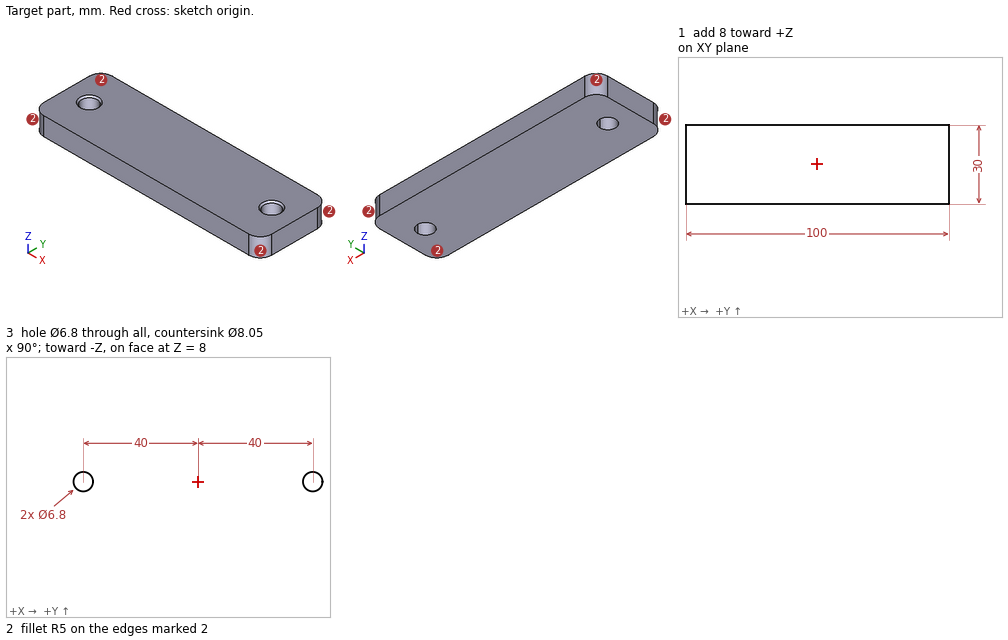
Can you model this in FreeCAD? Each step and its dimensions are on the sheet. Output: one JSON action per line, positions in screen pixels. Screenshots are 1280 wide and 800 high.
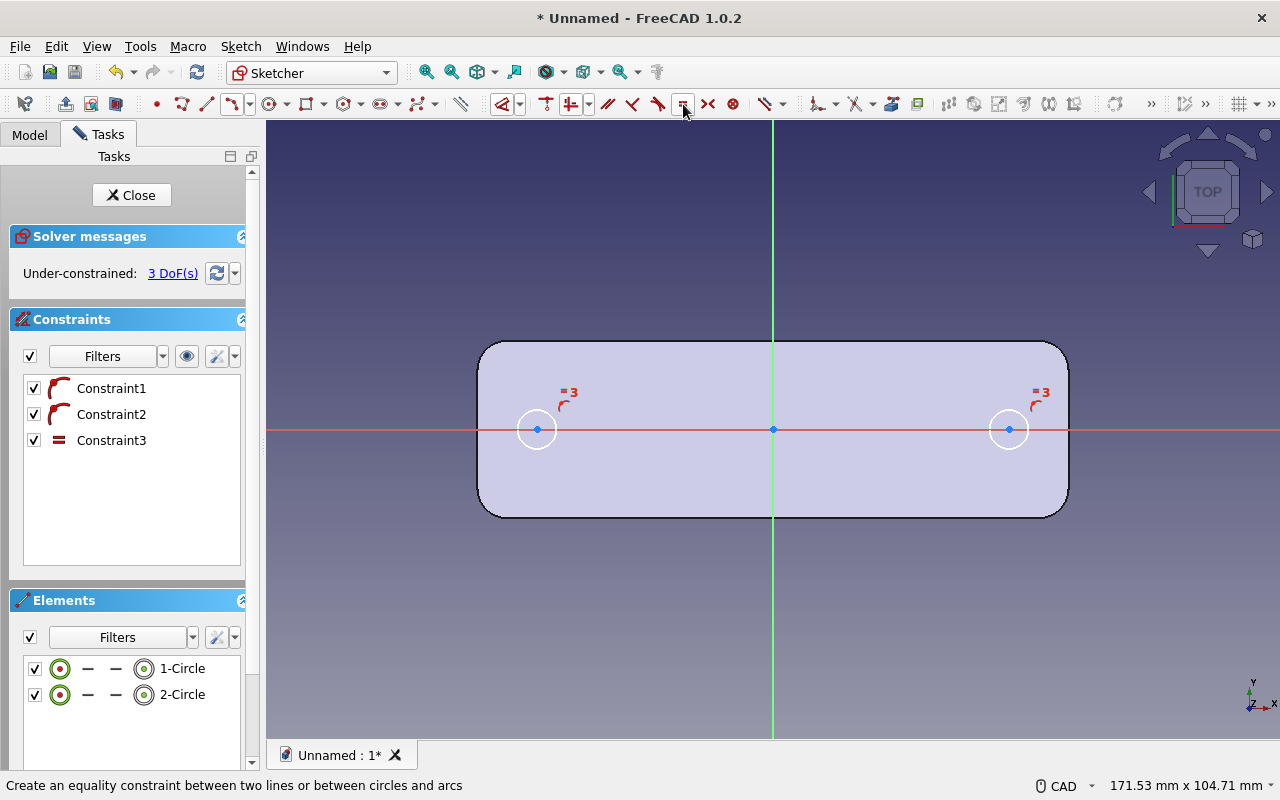
{"action": "left_click", "coordinate": [551, 416]}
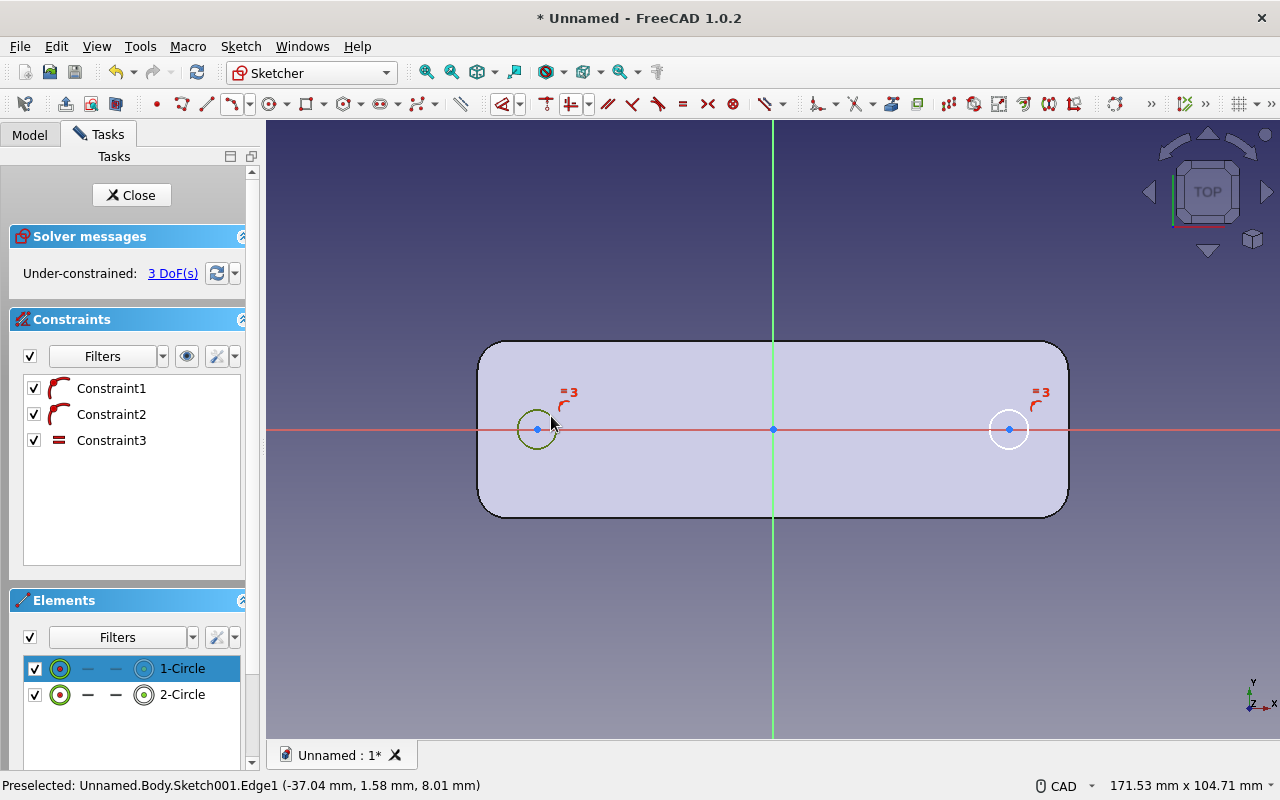
{"action": "key", "text": "k o"}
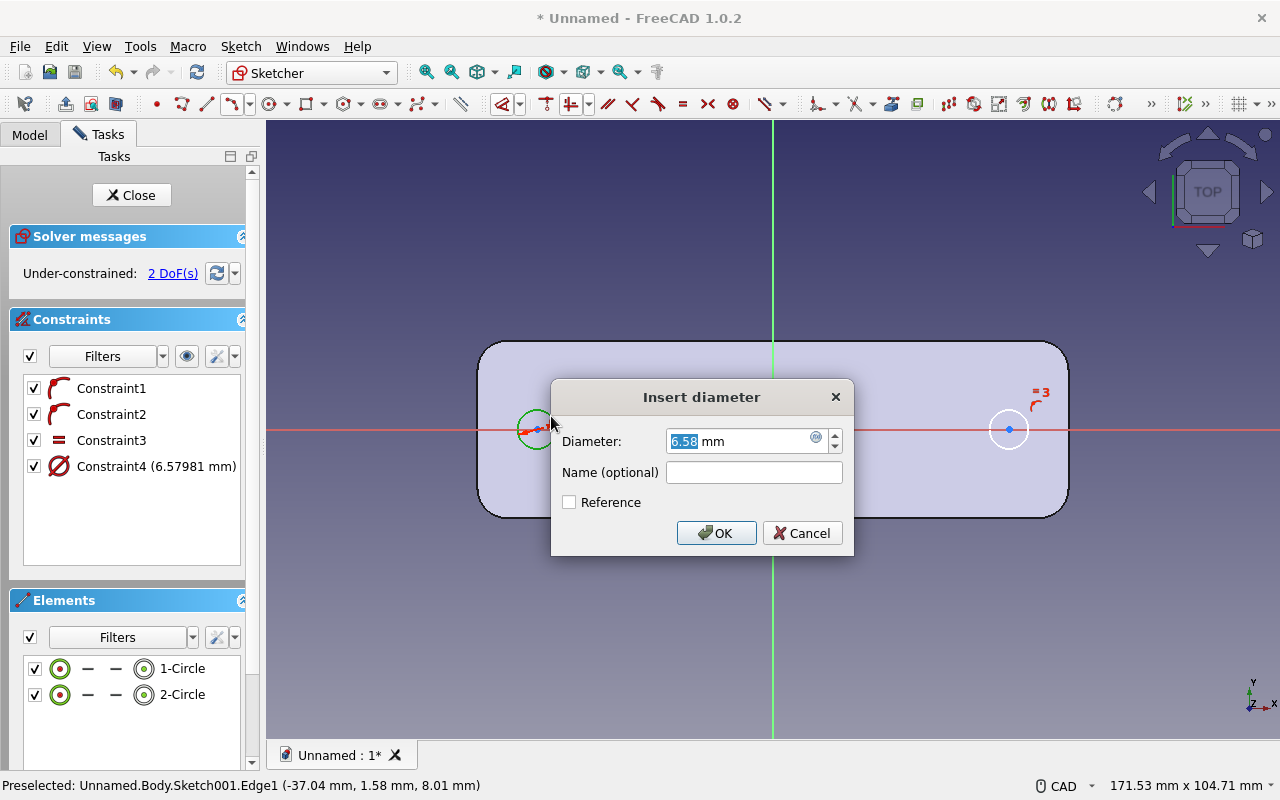
{"action": "type", "text": "6.8"}
{"action": "key", "text": "Return"}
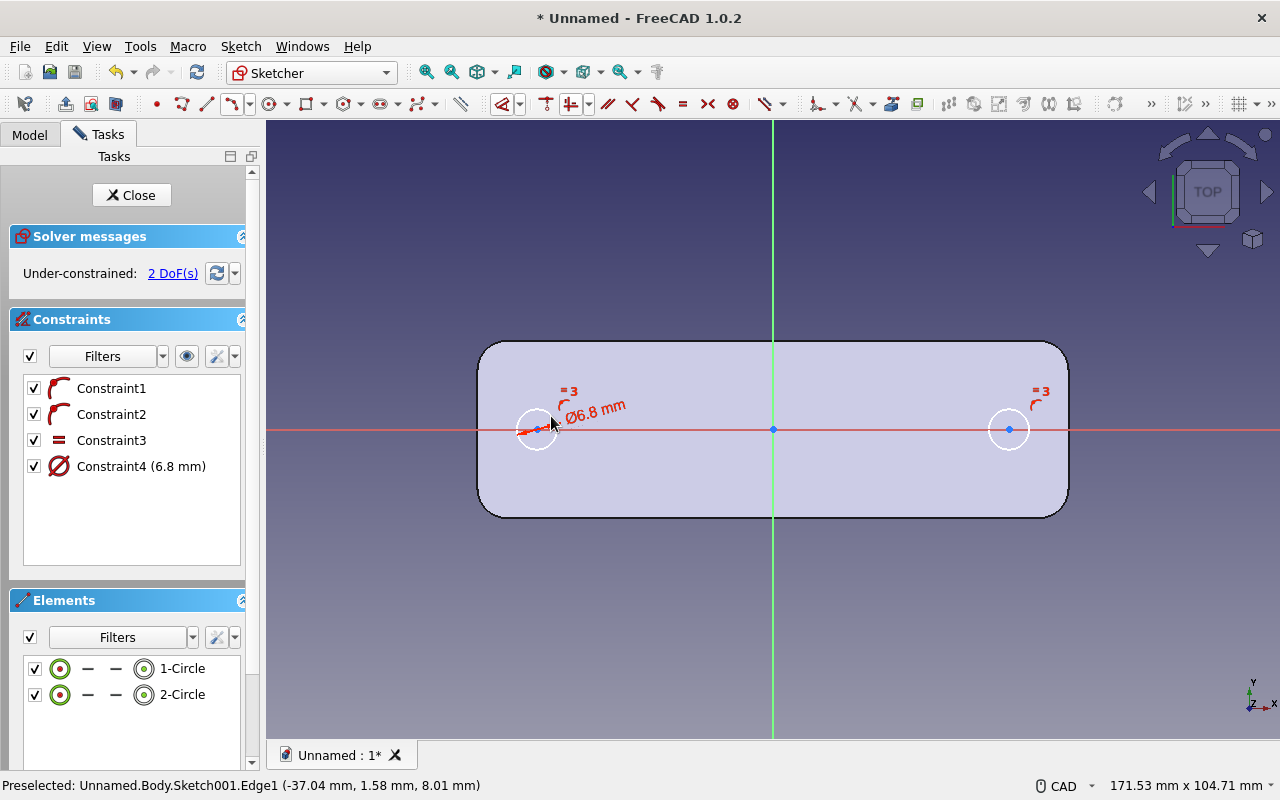
{"action": "left_click", "coordinate": [537, 430]}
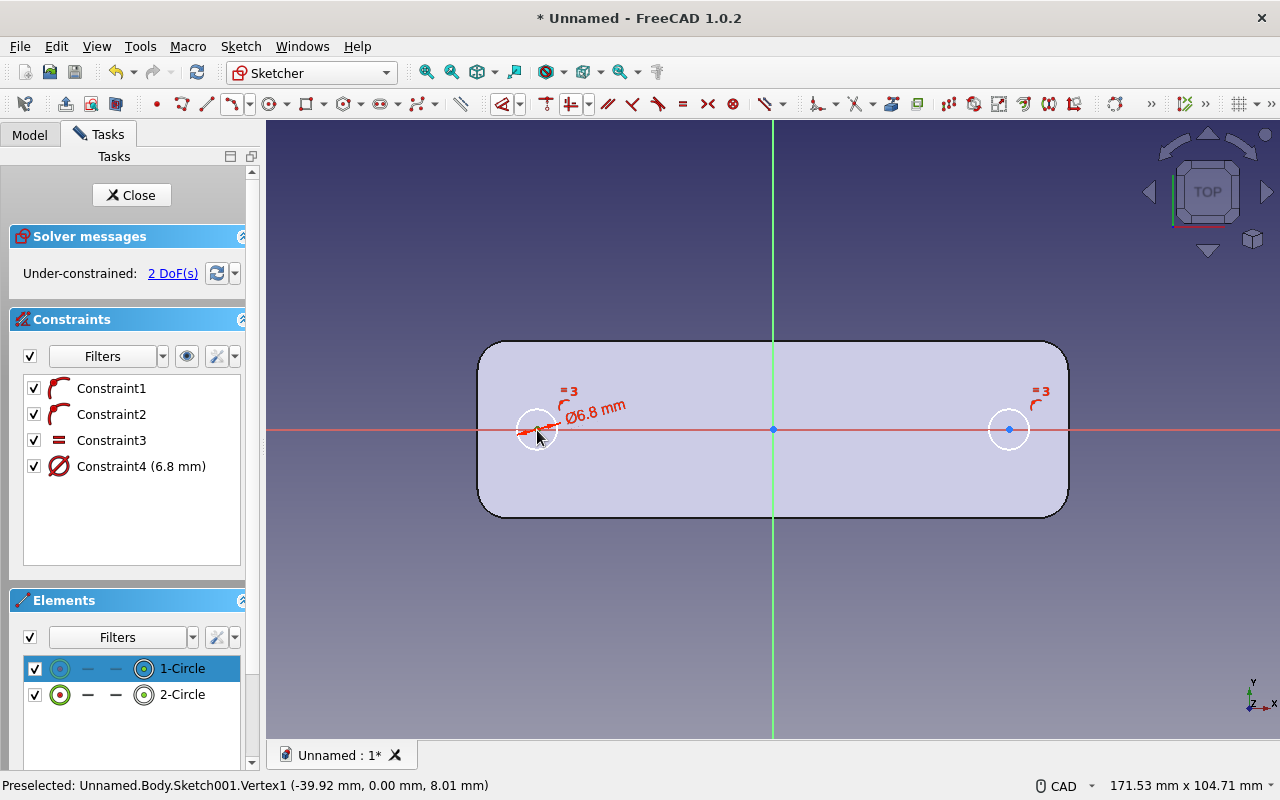
{"action": "left_click", "coordinate": [520, 104]}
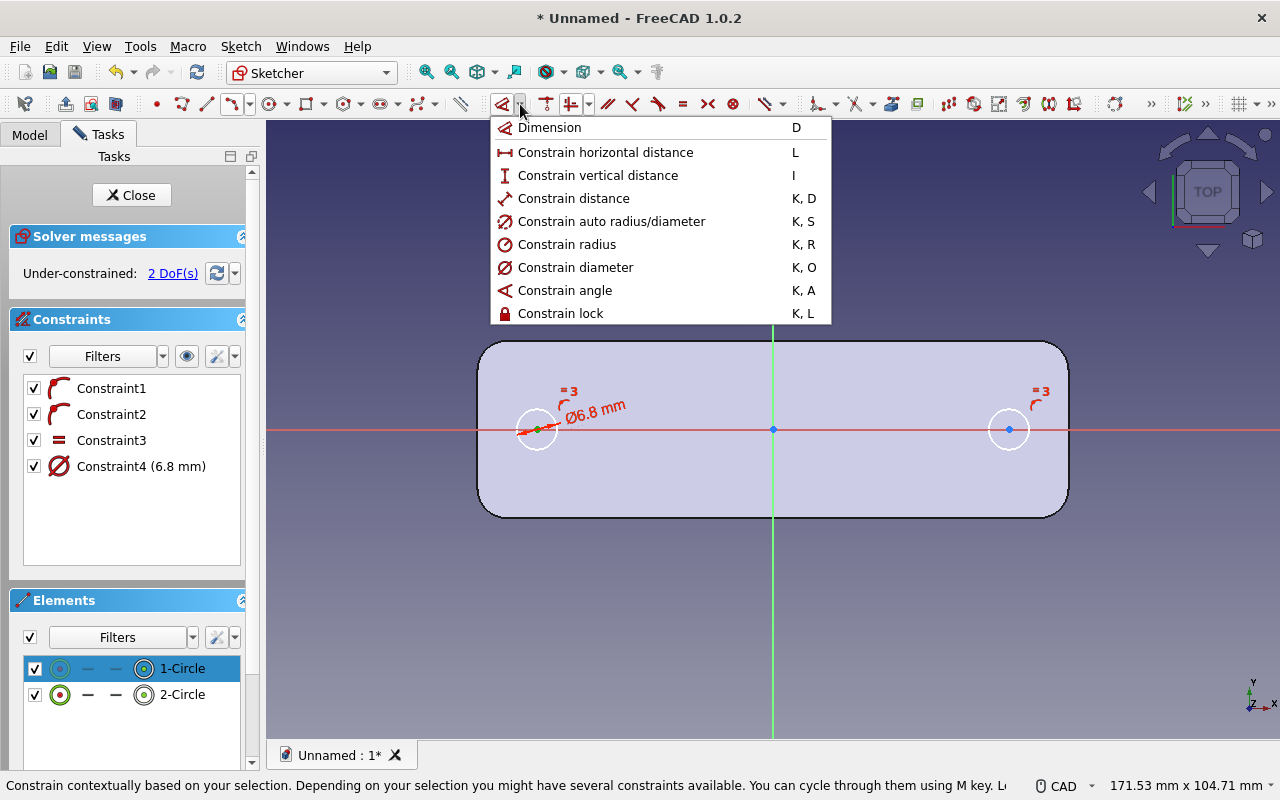
{"action": "left_click", "coordinate": [661, 152]}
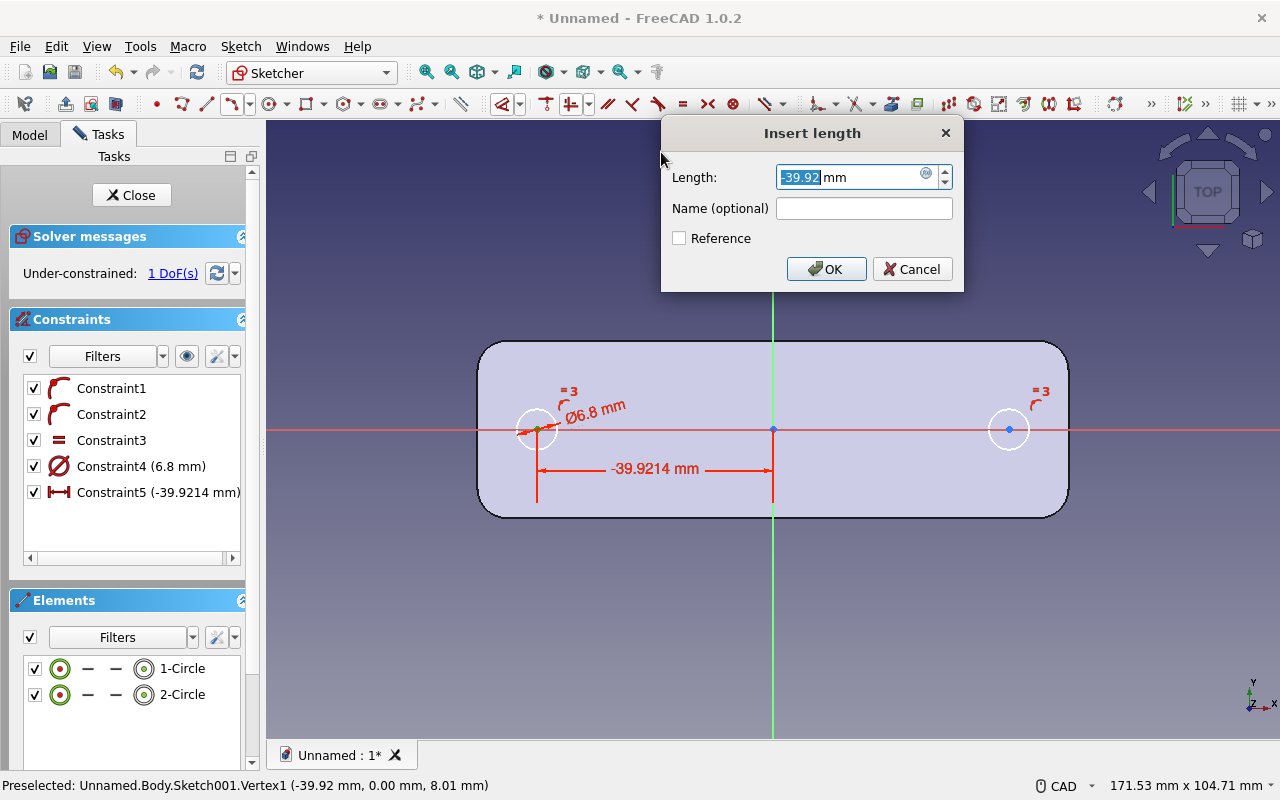
{"action": "type", "text": "-40"}
{"action": "key", "text": "Return"}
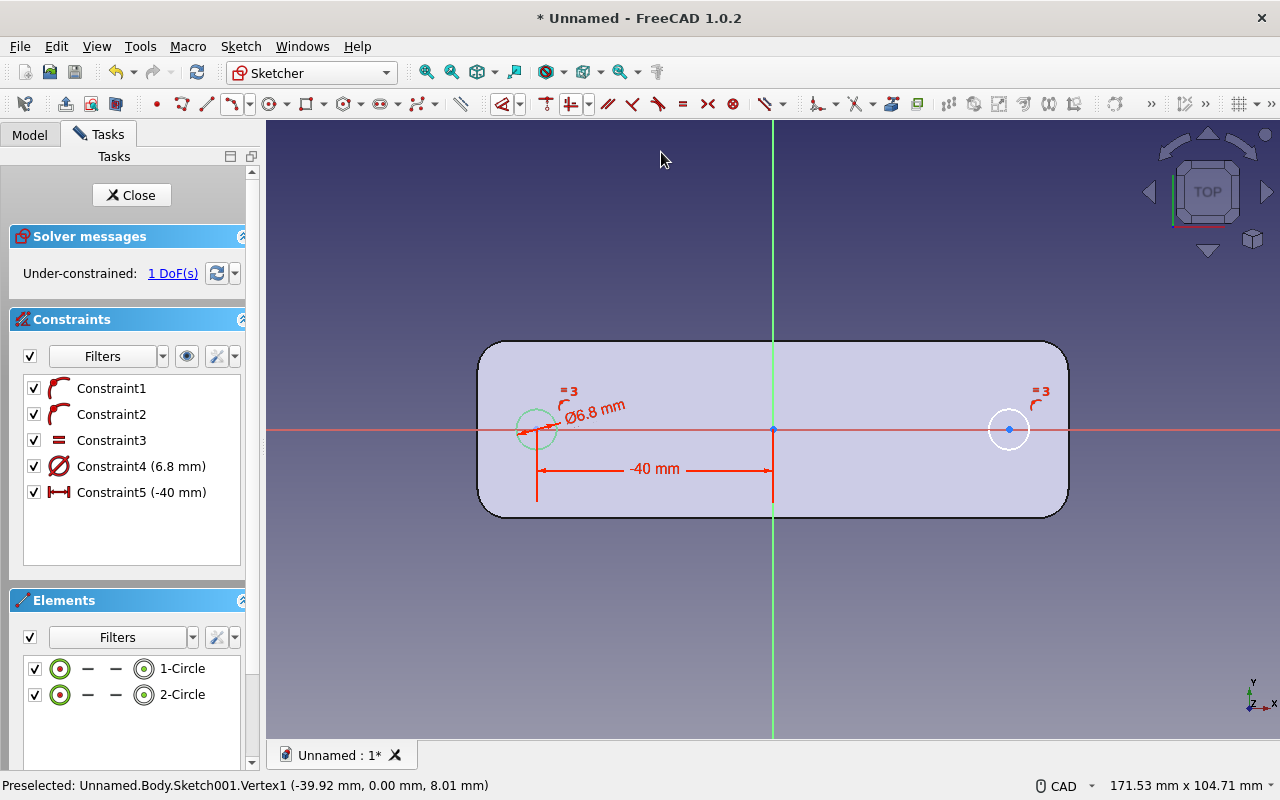
{"action": "left_click", "coordinate": [1009, 430]}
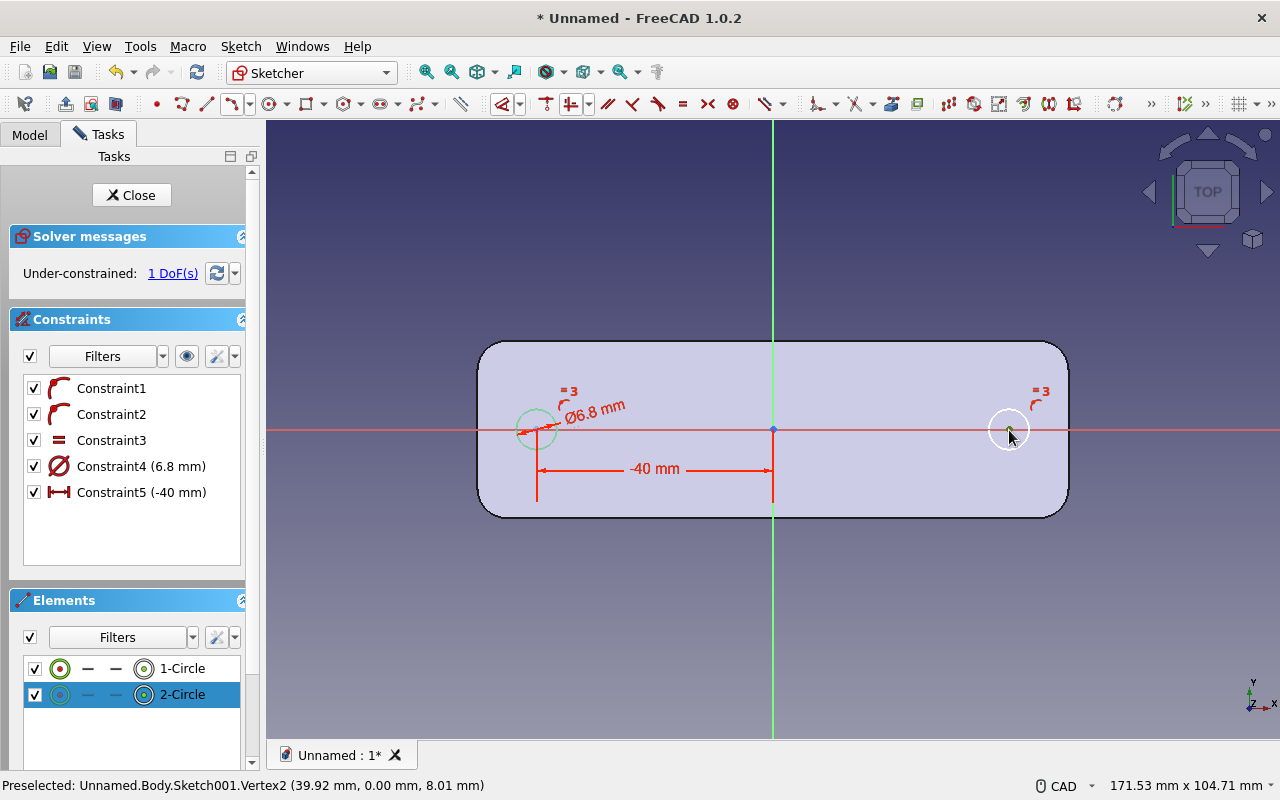
{"action": "left_click", "coordinate": [520, 104]}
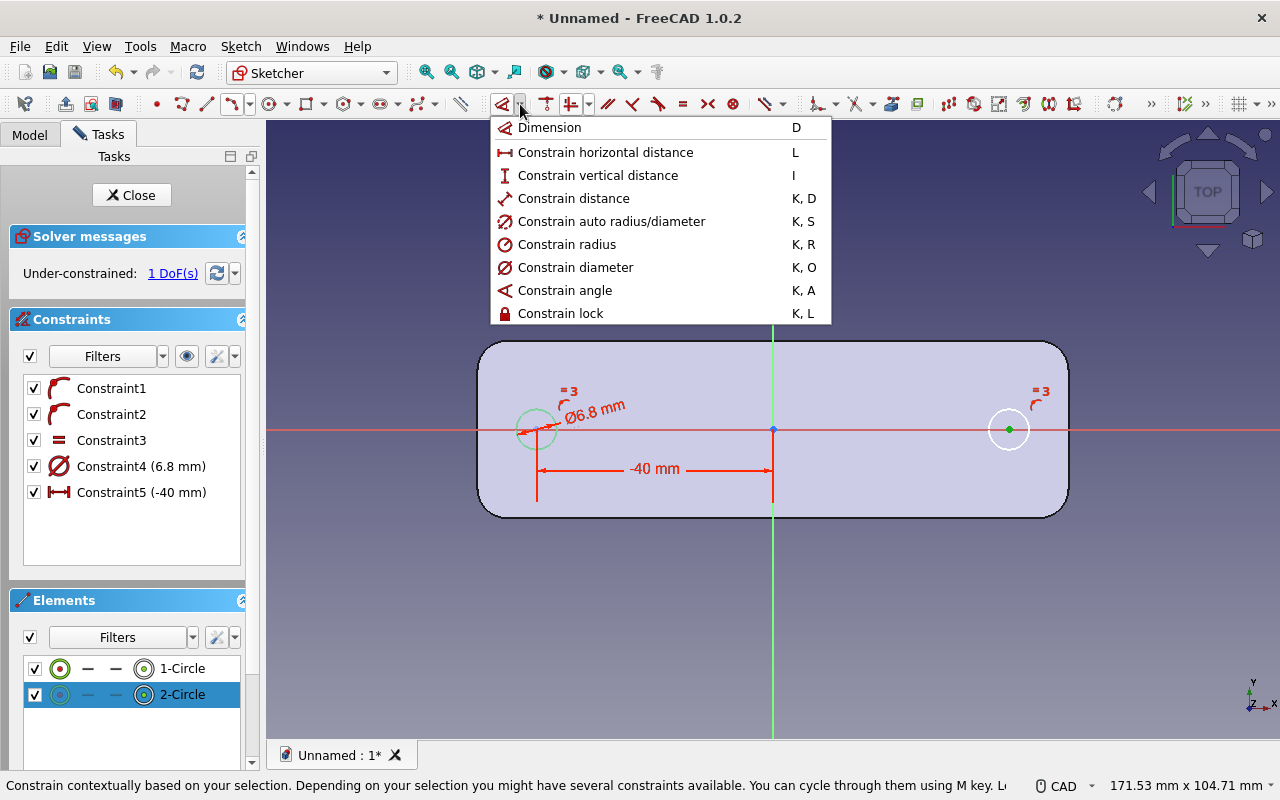
{"action": "left_click", "coordinate": [661, 152]}